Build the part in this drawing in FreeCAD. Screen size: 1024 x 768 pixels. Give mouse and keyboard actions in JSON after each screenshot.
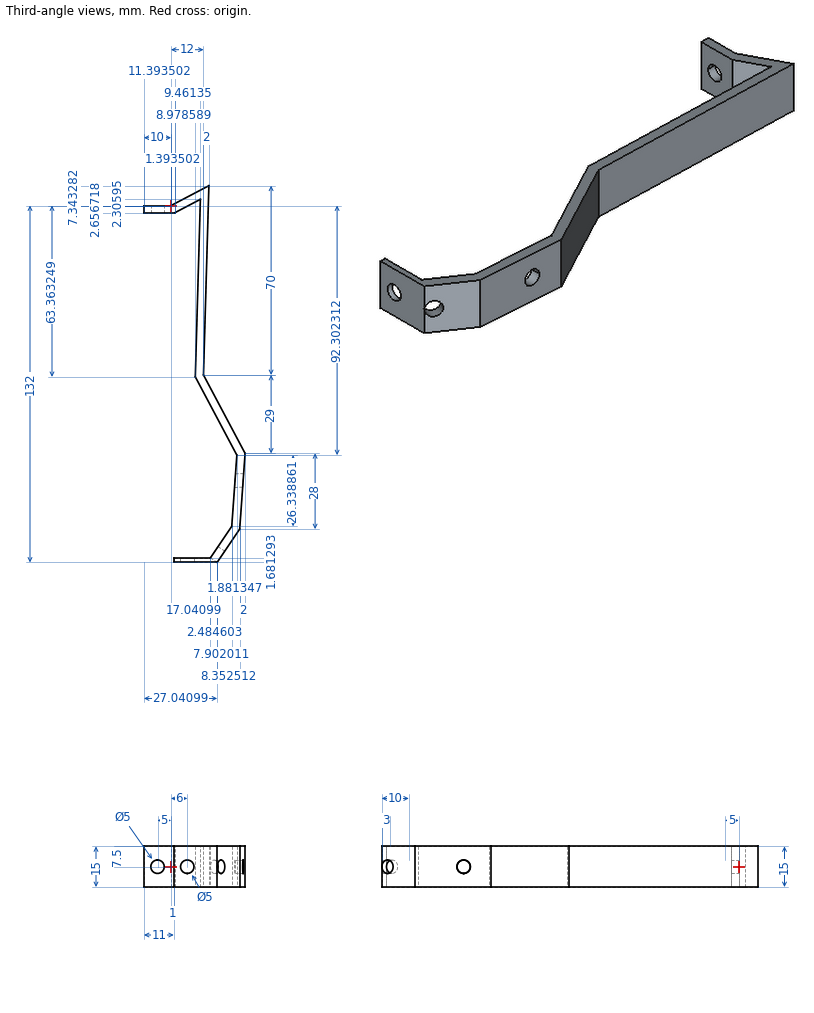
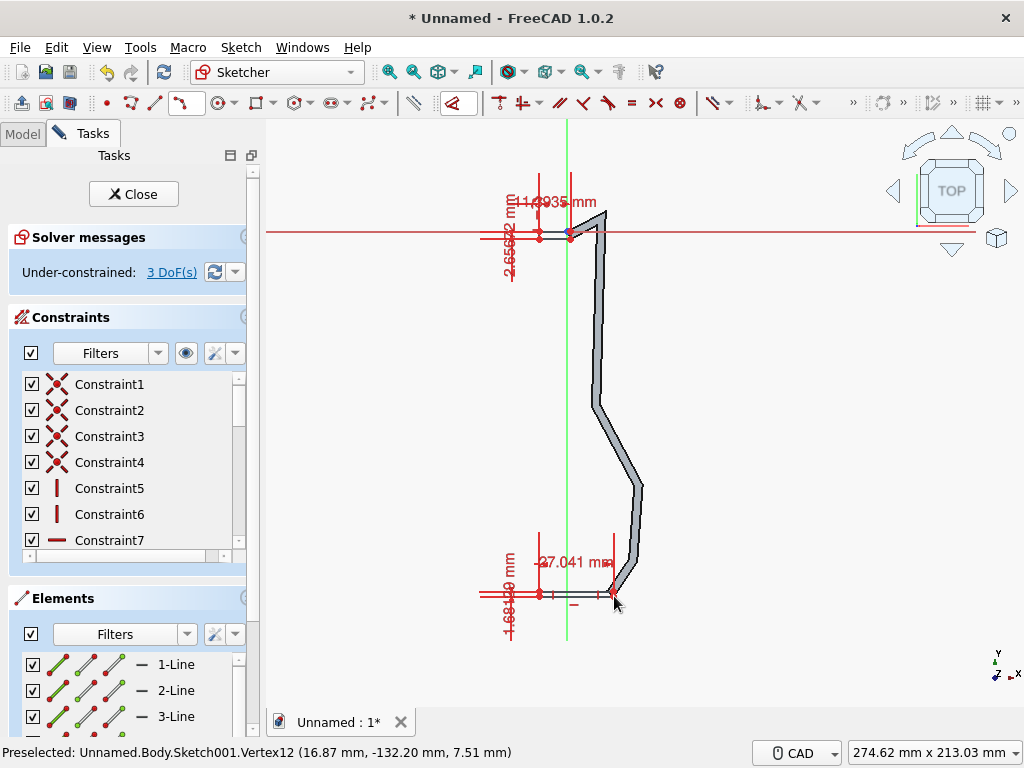
{"action": "scroll", "coordinate": [539, 232], "scroll_direction": "up", "scroll_amount": 3}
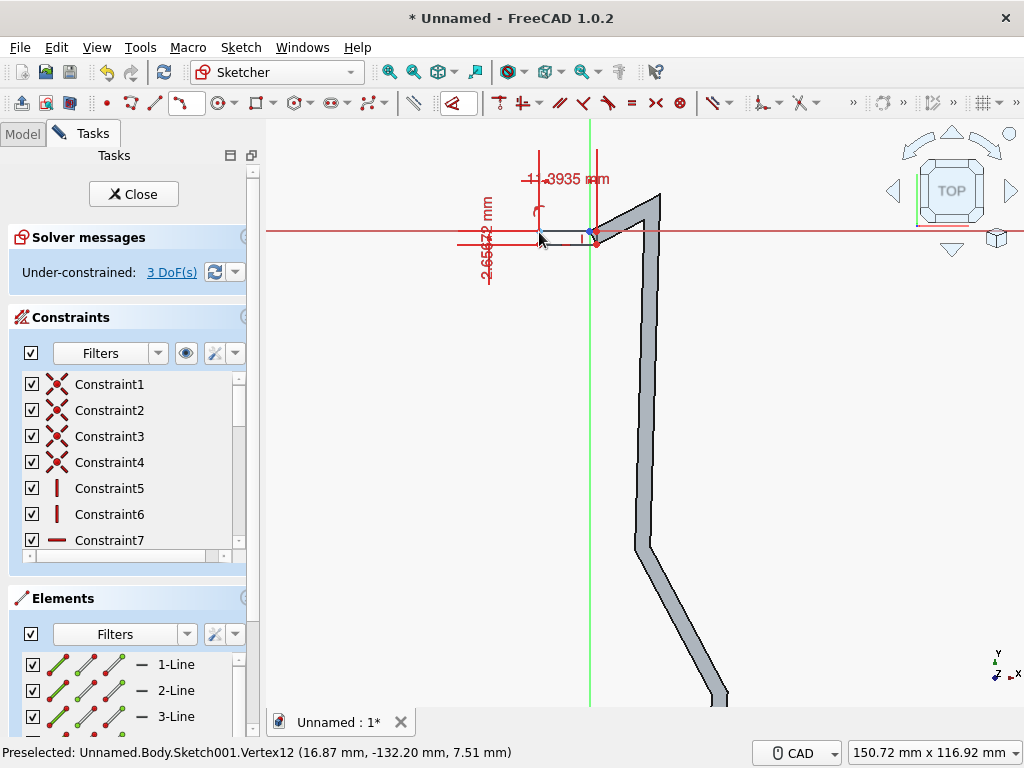
{"action": "left_click", "coordinate": [539, 231]}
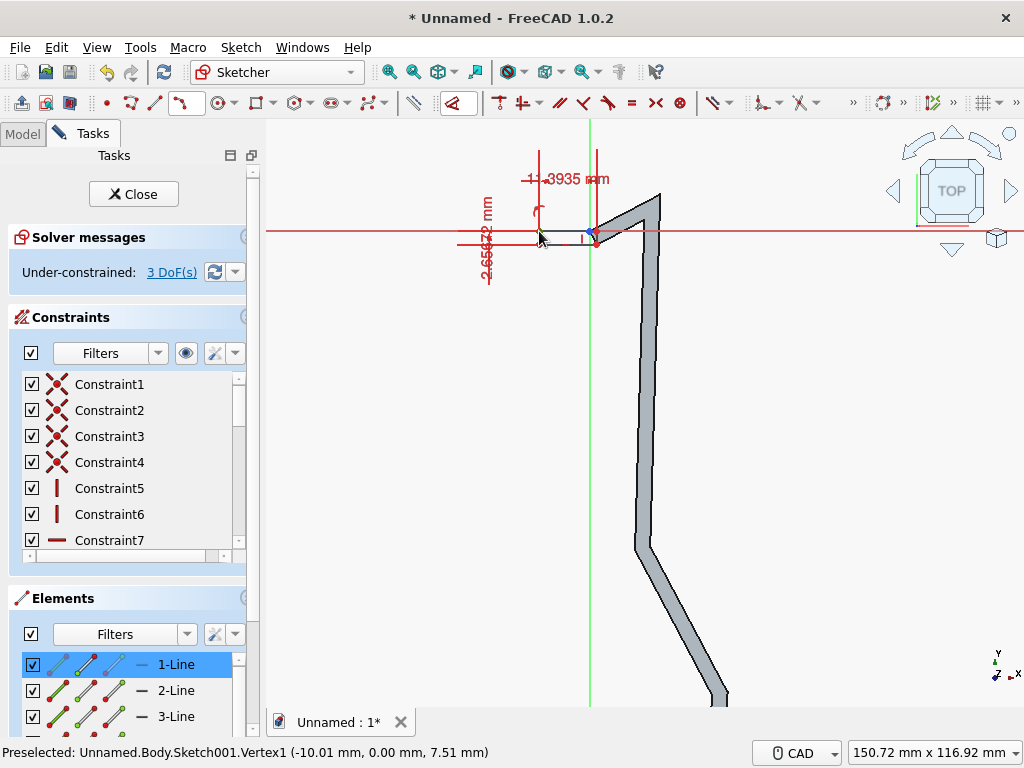
{"action": "left_click", "coordinate": [472, 104]}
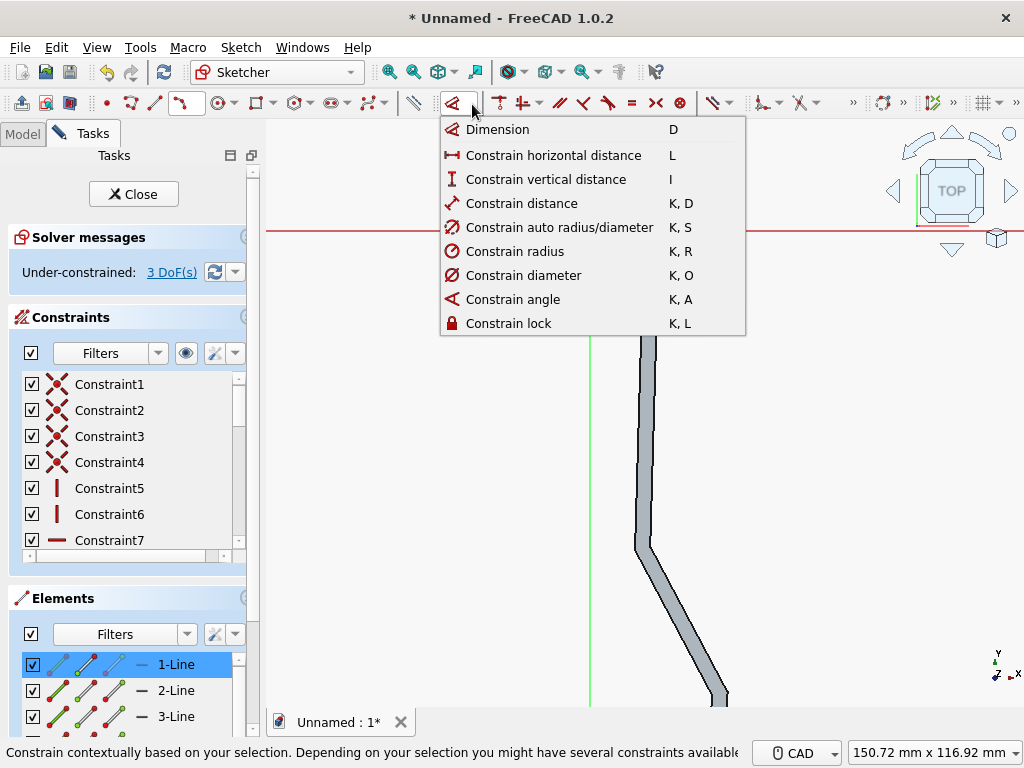
{"action": "left_click", "coordinate": [593, 155]}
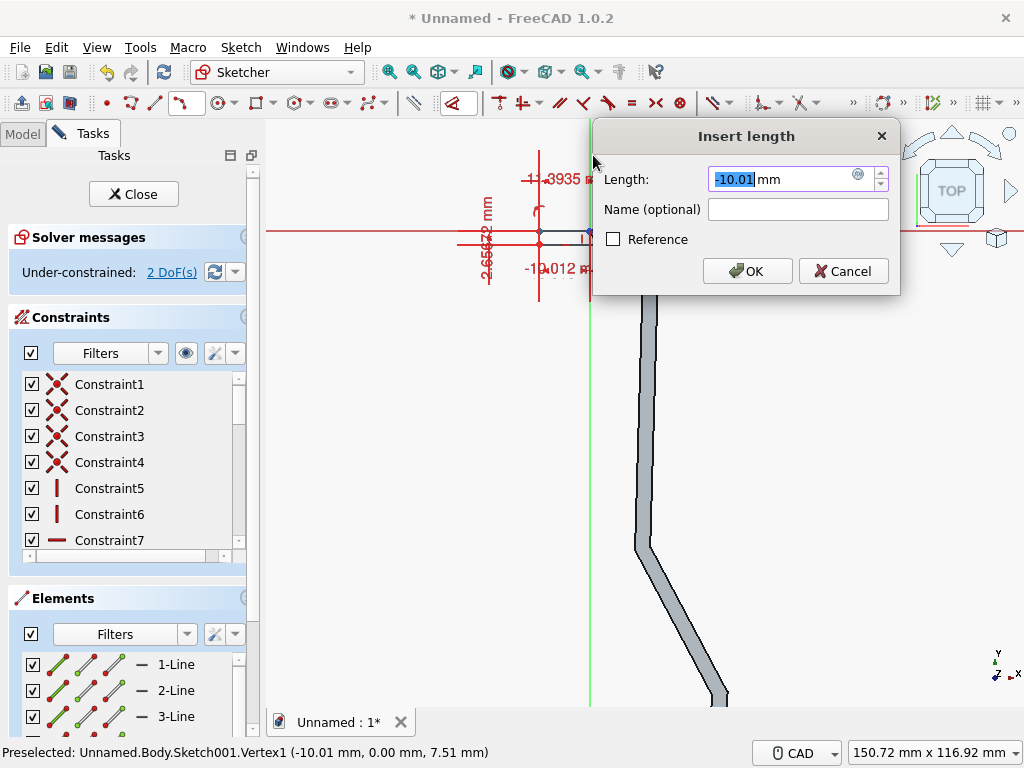
{"action": "type", "text": "-10"}
{"action": "key", "text": "Return"}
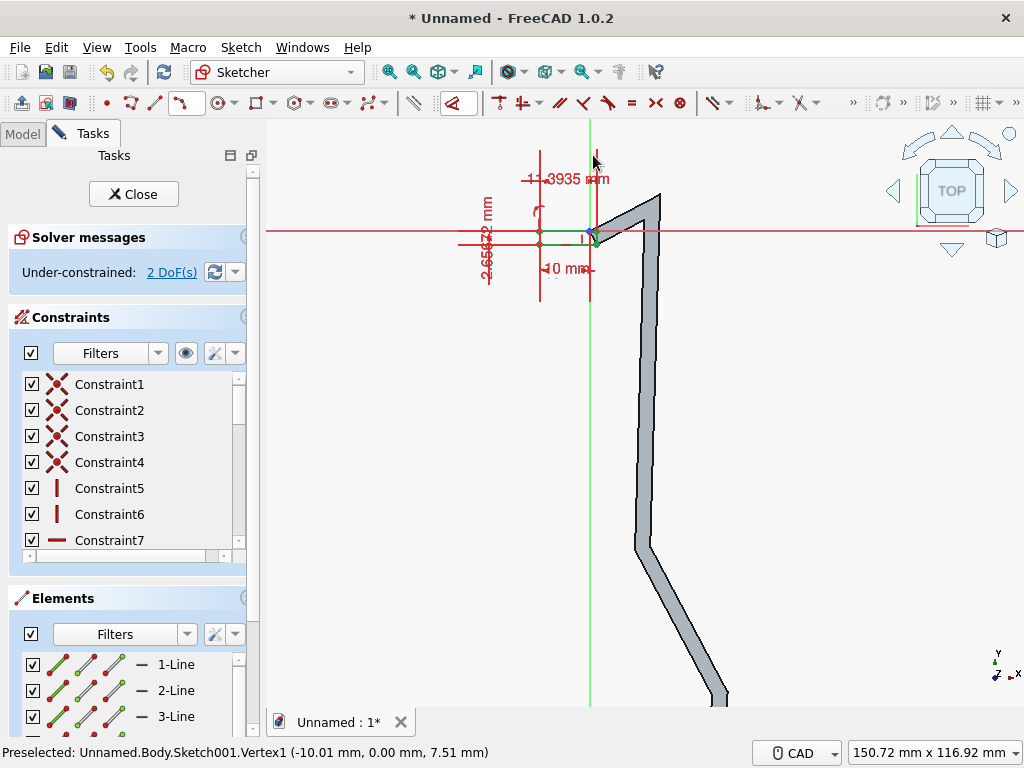
{"action": "scroll", "coordinate": [539, 230], "scroll_direction": "down", "scroll_amount": 3}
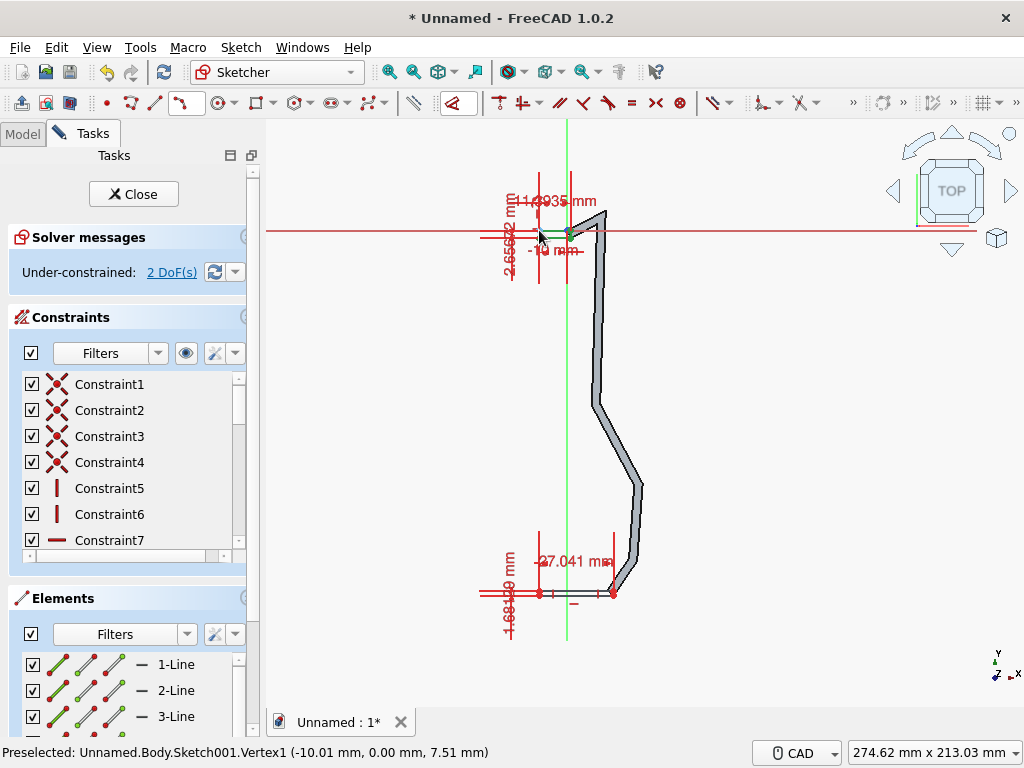
{"action": "scroll", "coordinate": [539, 591], "scroll_direction": "up", "scroll_amount": 5}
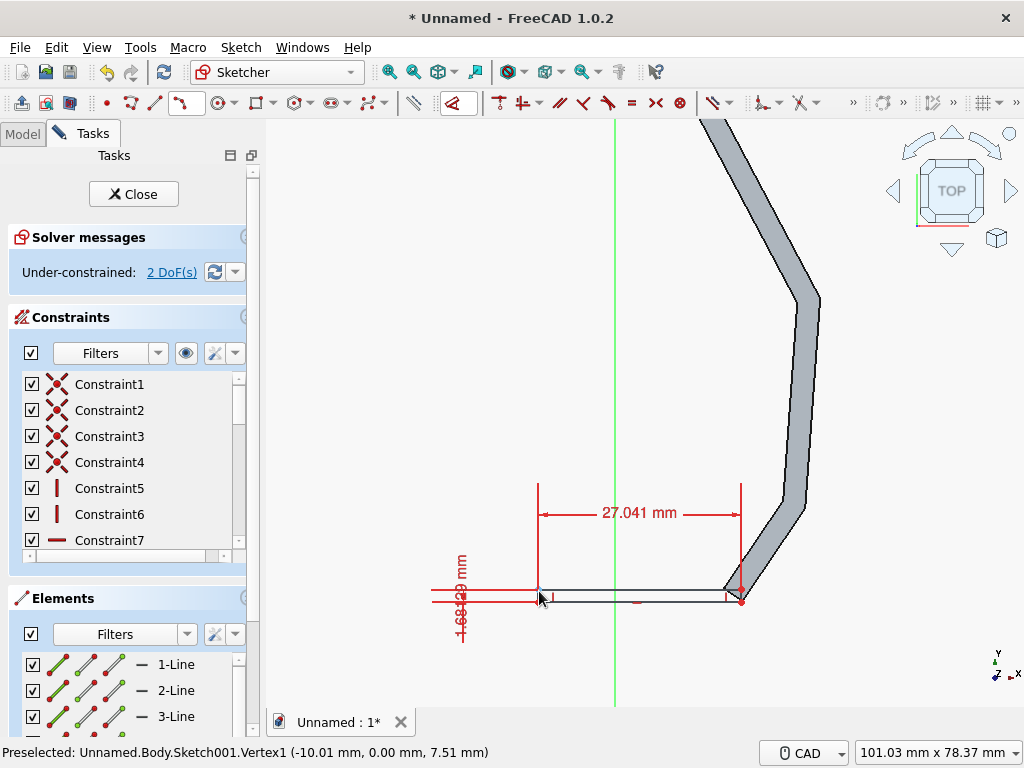
{"action": "left_click", "coordinate": [538, 590]}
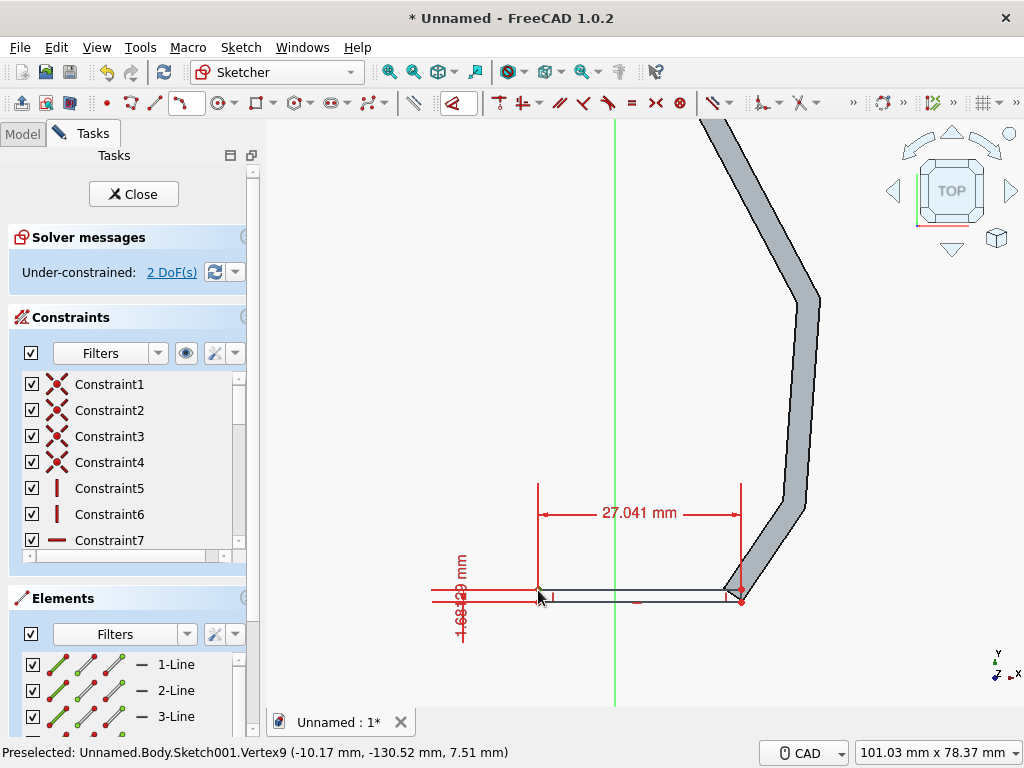
{"action": "left_click", "coordinate": [472, 104]}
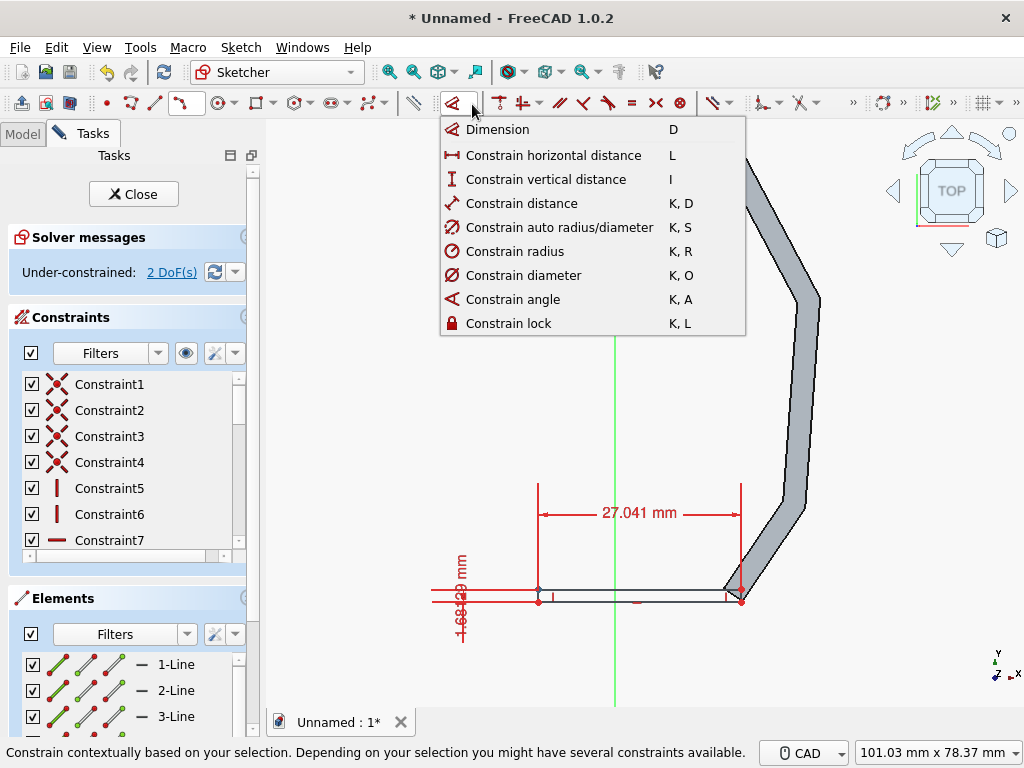
{"action": "left_click", "coordinate": [593, 155]}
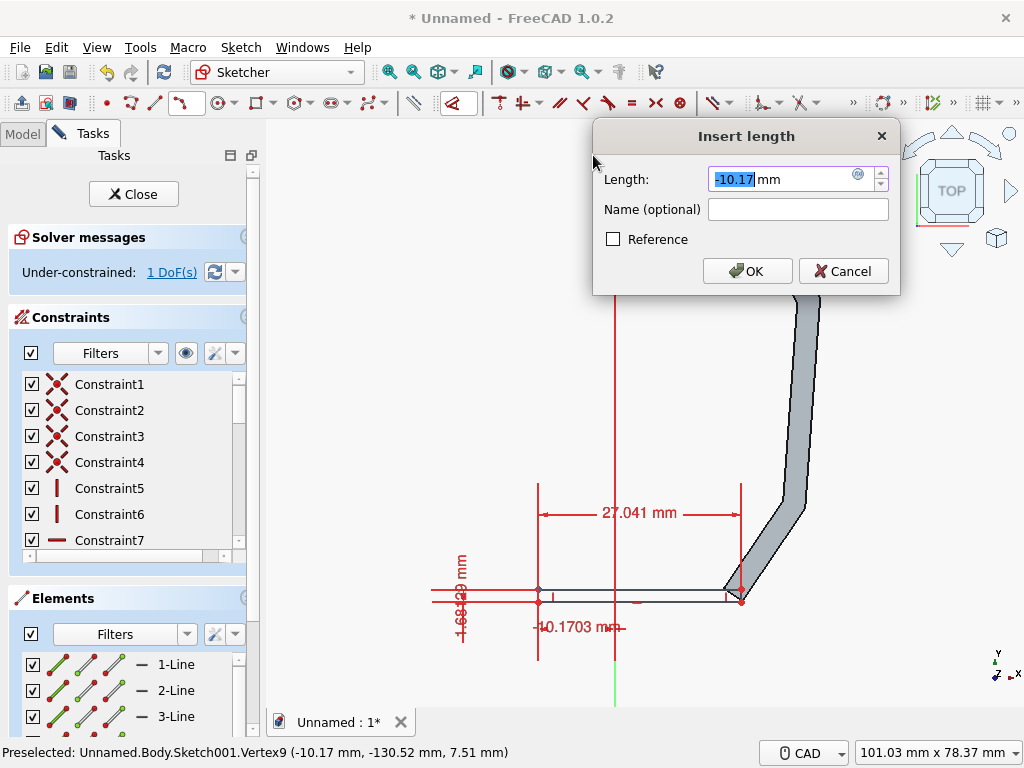
{"action": "type", "text": "-10"}
{"action": "key", "text": "Return"}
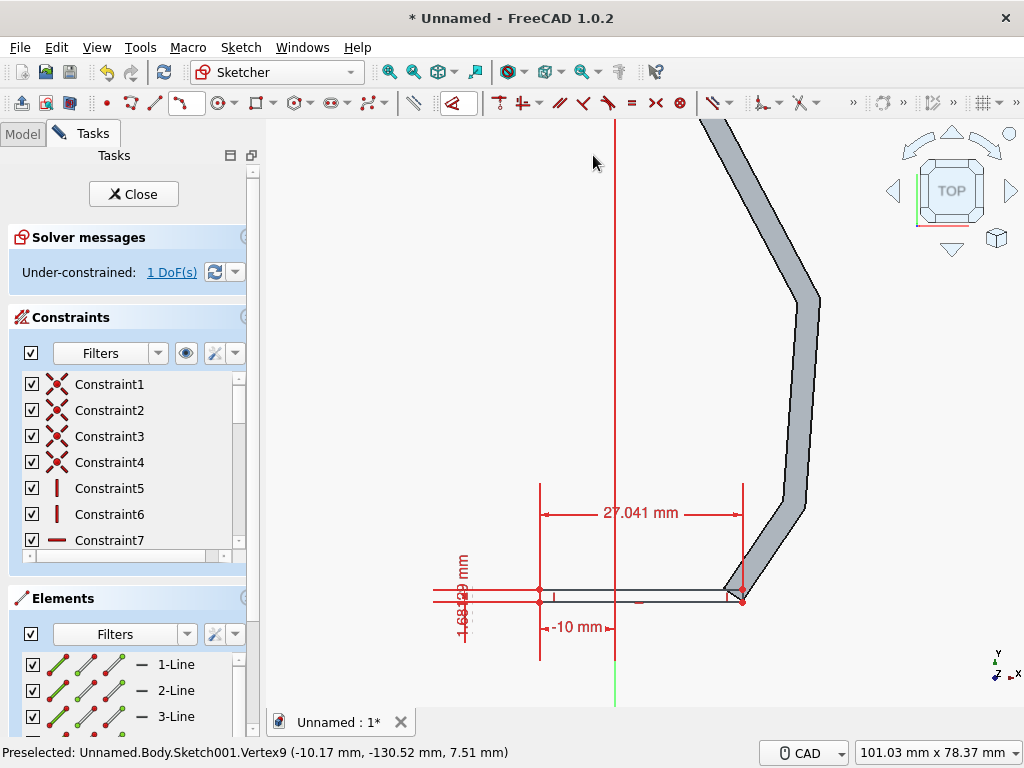
{"action": "left_click", "coordinate": [540, 602]}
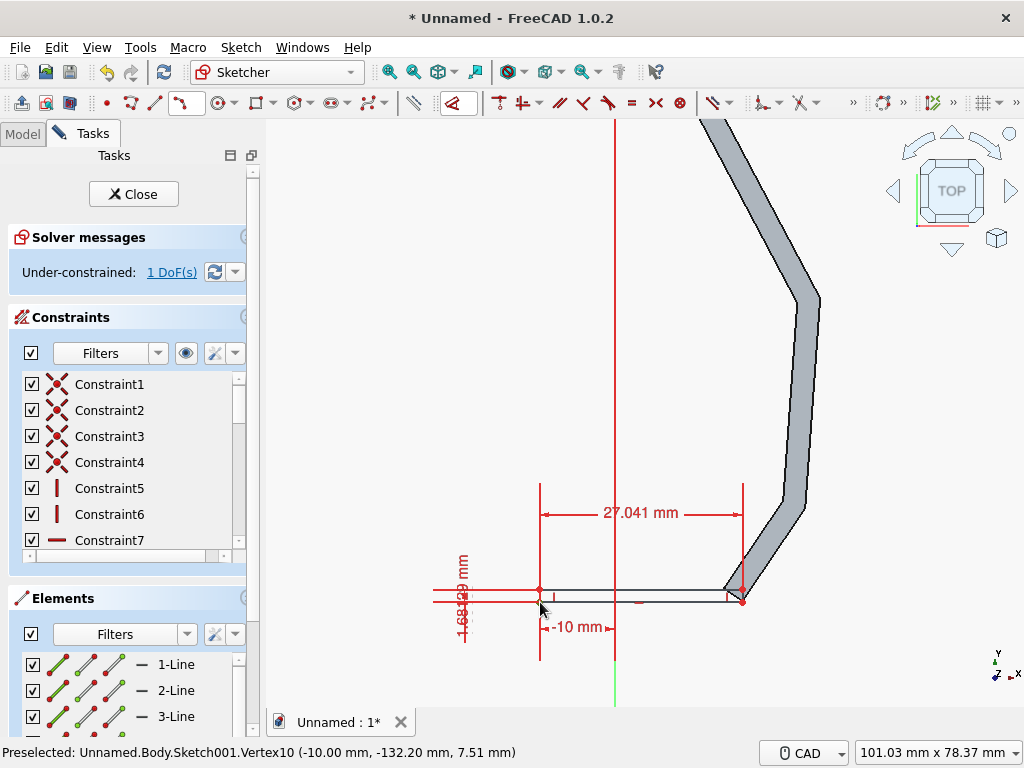
{"action": "key", "text": "i"}